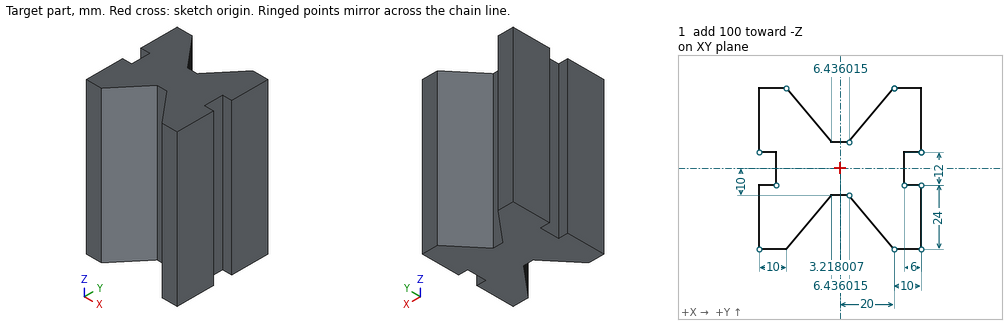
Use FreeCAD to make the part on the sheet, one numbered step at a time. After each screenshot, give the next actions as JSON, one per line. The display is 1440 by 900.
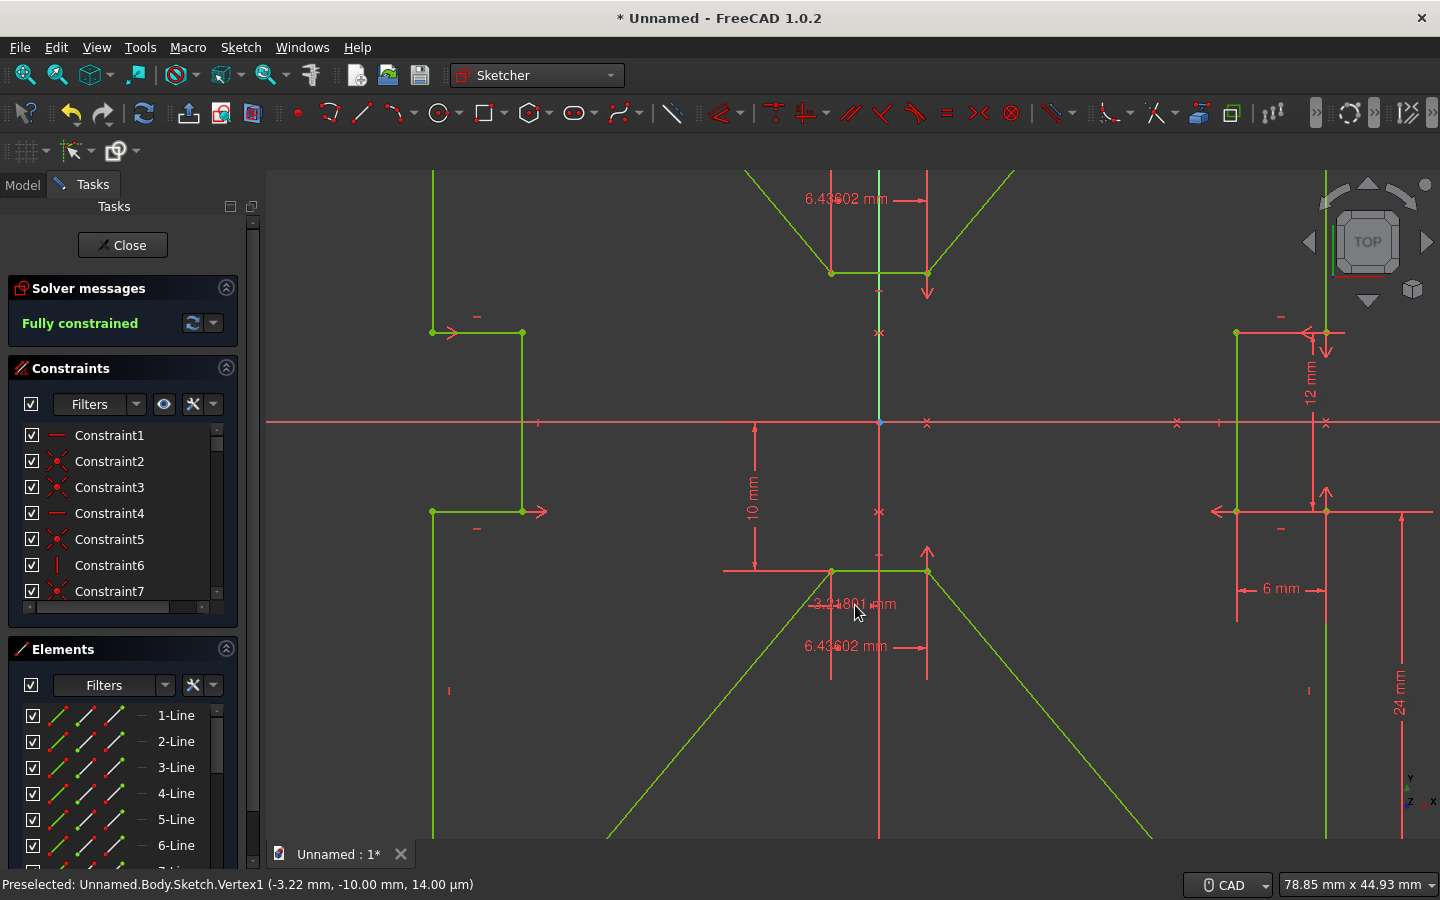
{"action": "left_click", "coordinate": [123, 245]}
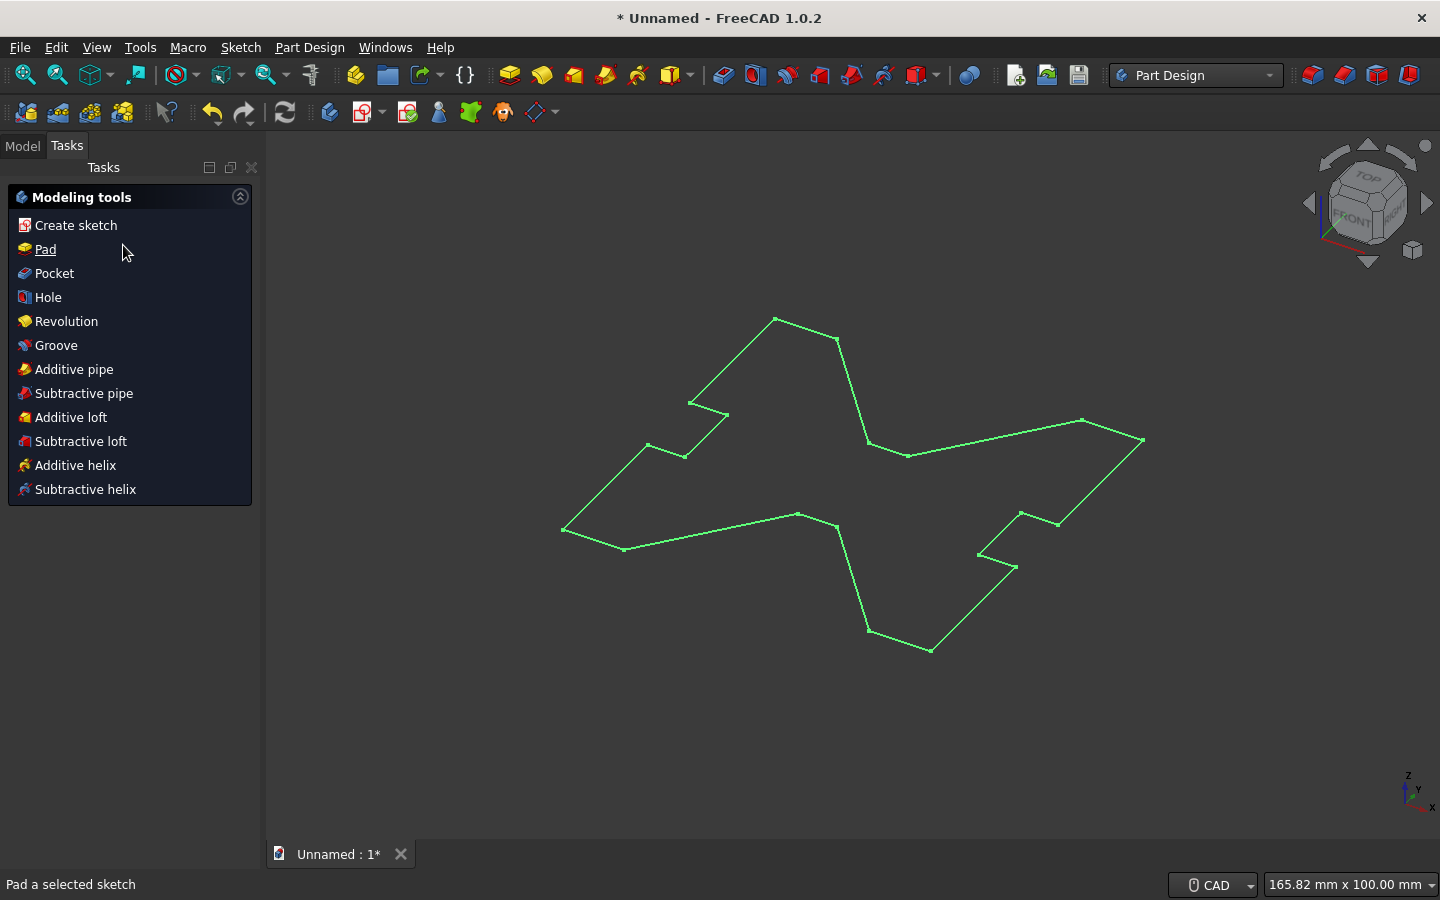
{"action": "left_click", "coordinate": [510, 76]}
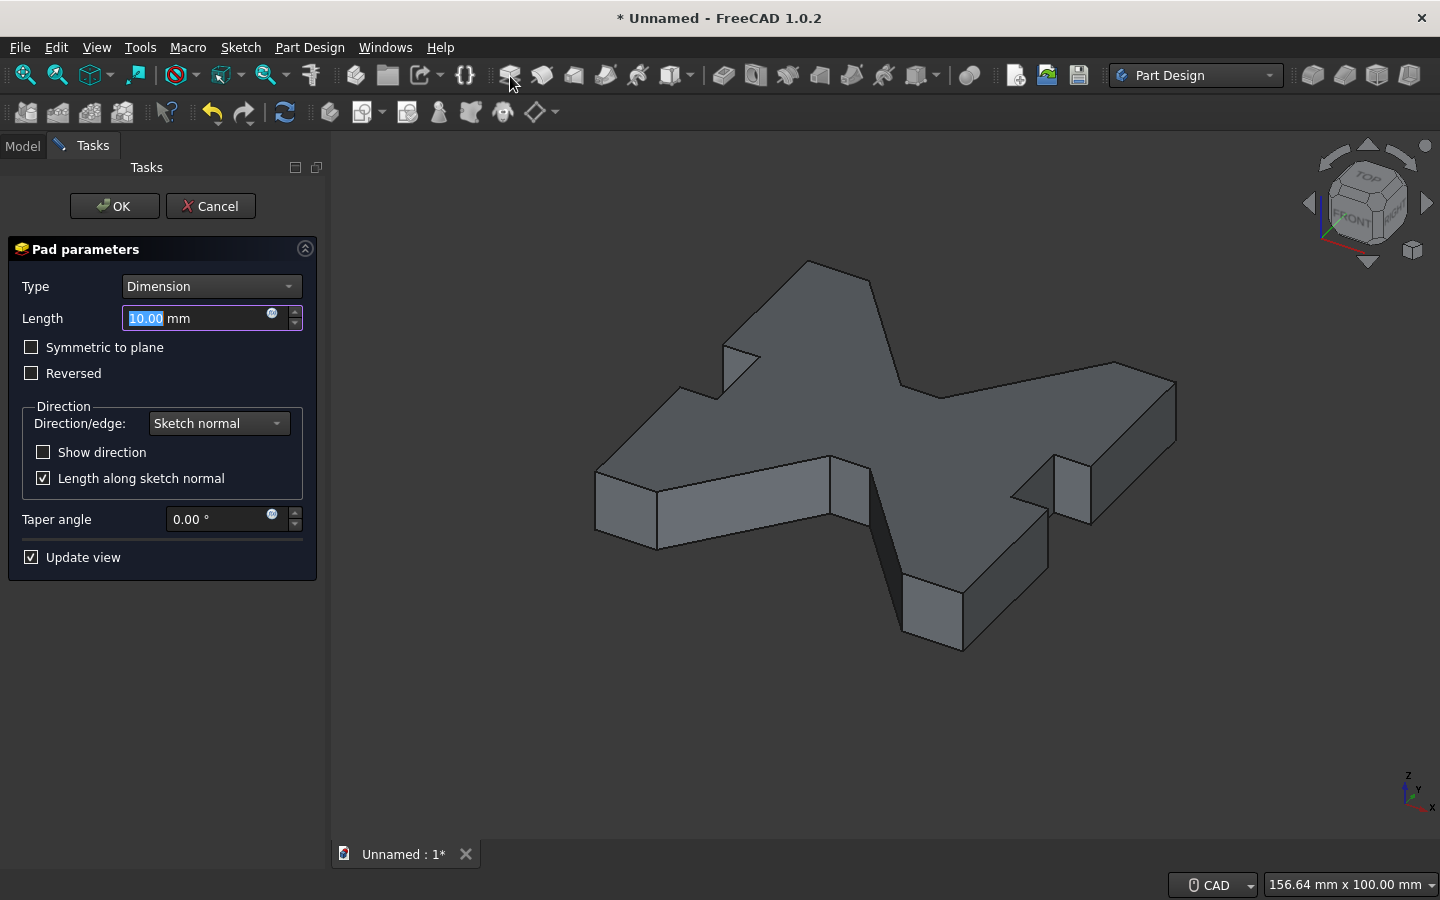
{"action": "type", "text": "100"}
{"action": "key", "text": "Tab"}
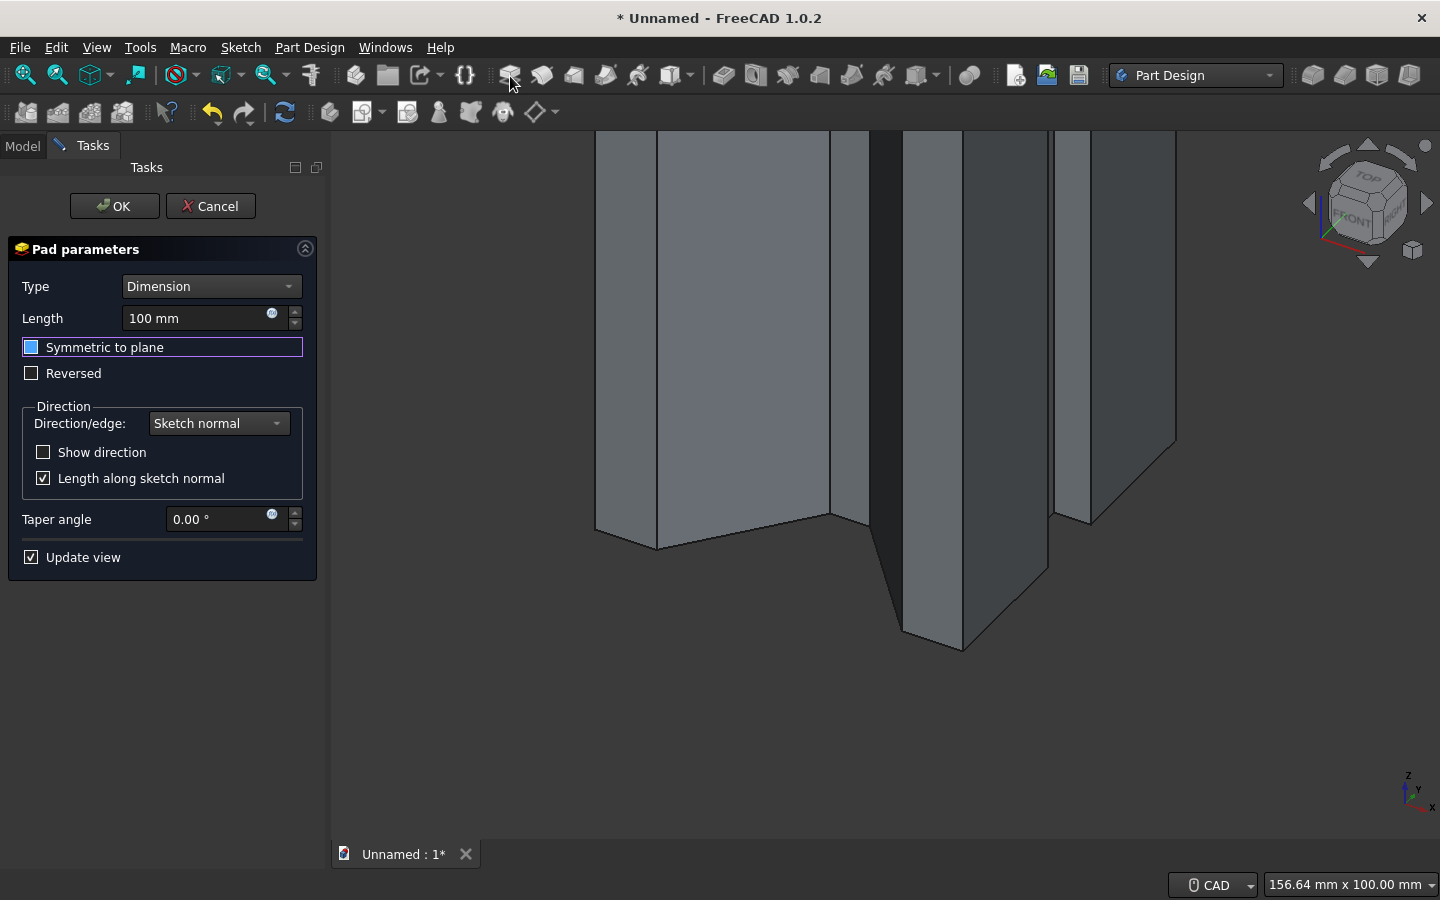
{"action": "left_click", "coordinate": [30, 373]}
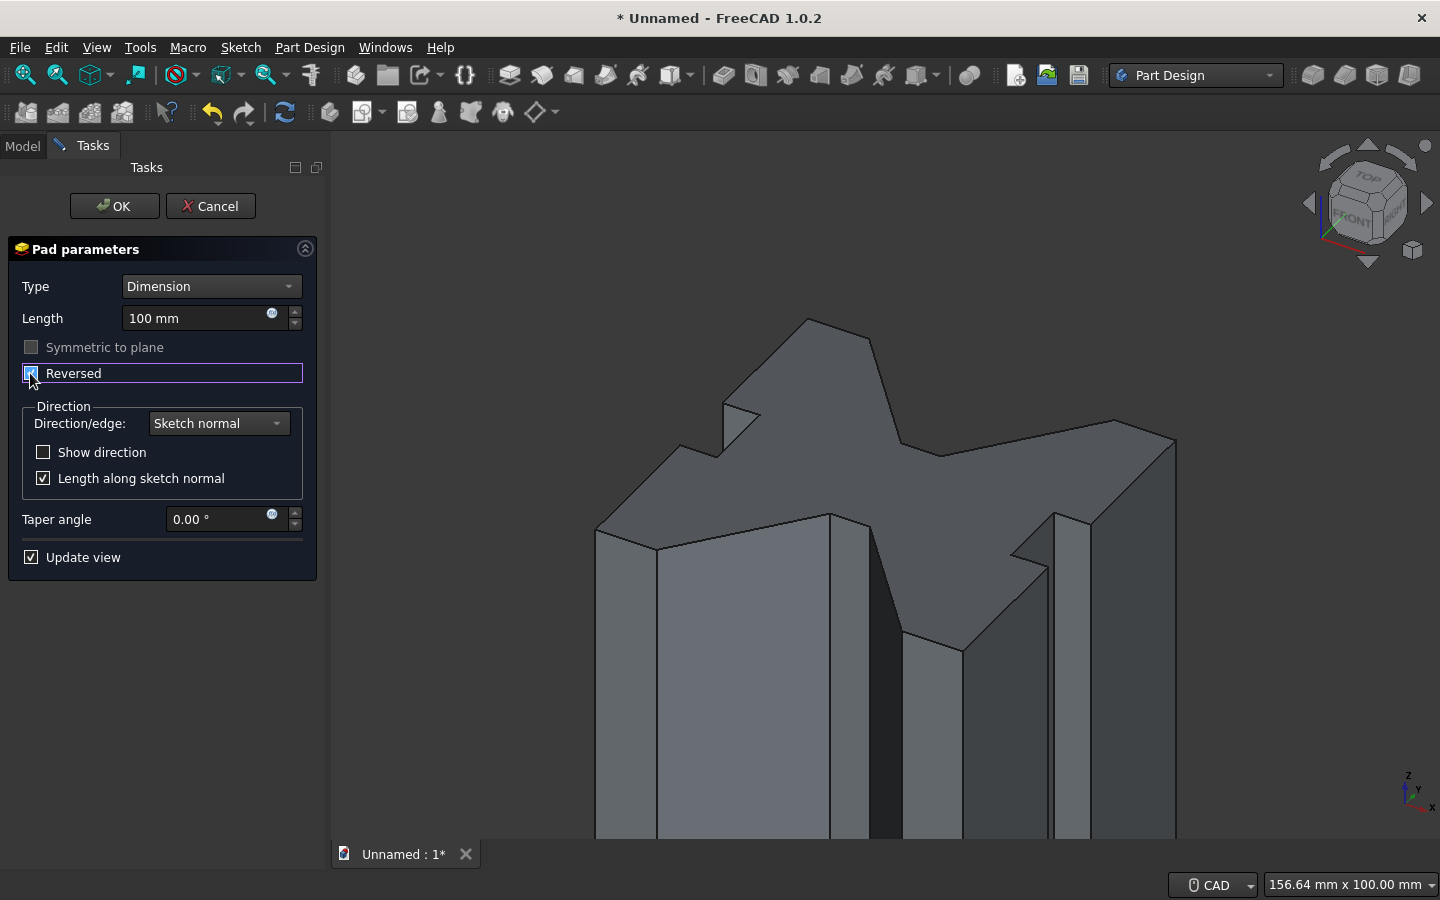
{"action": "left_click", "coordinate": [115, 206]}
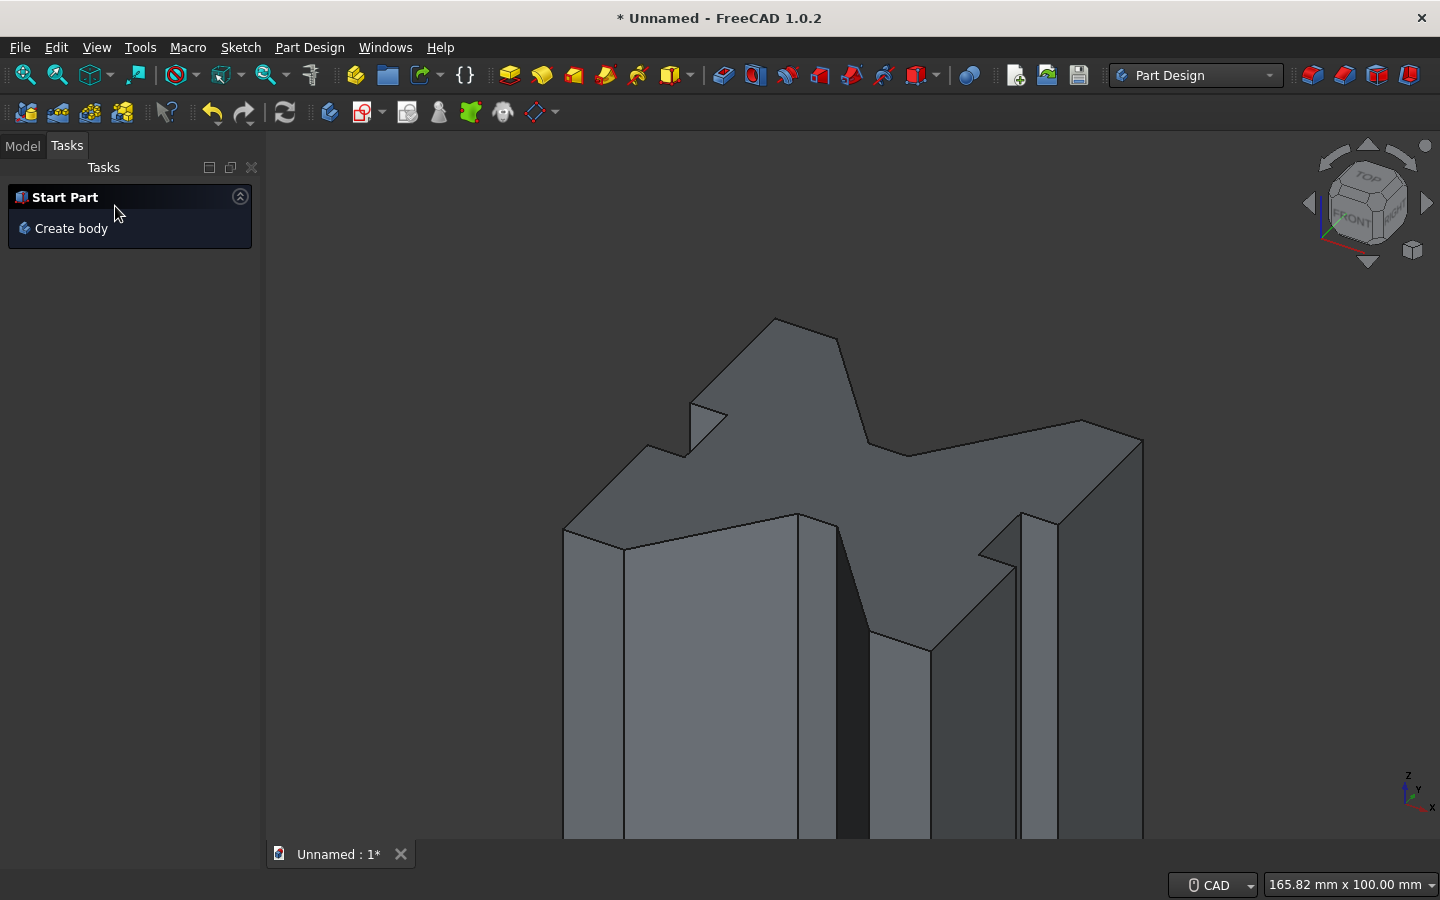
{"action": "key", "text": "0"}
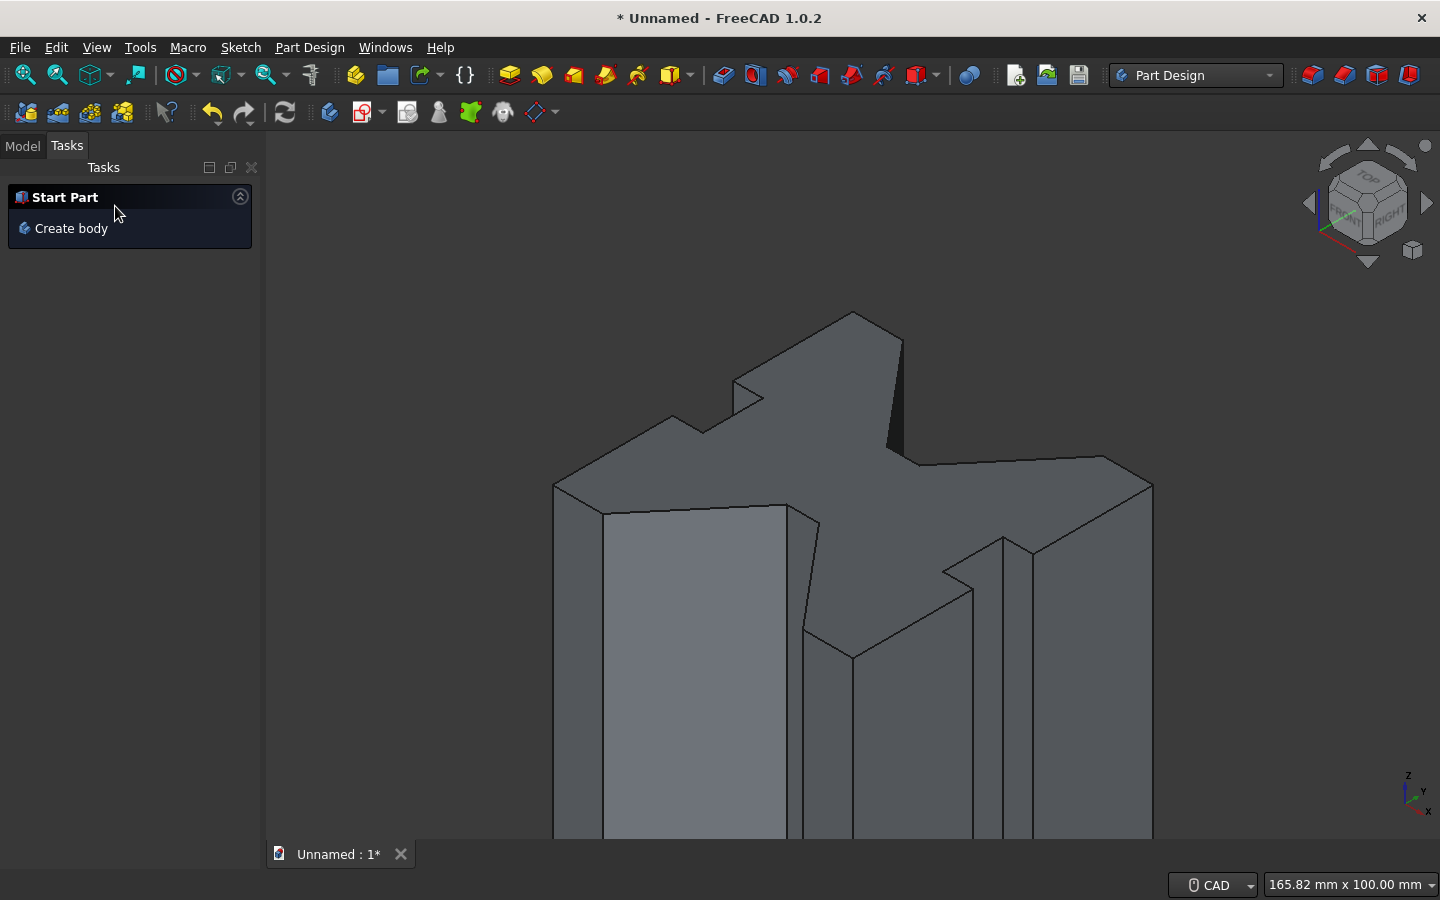
{"action": "key", "text": "v f"}